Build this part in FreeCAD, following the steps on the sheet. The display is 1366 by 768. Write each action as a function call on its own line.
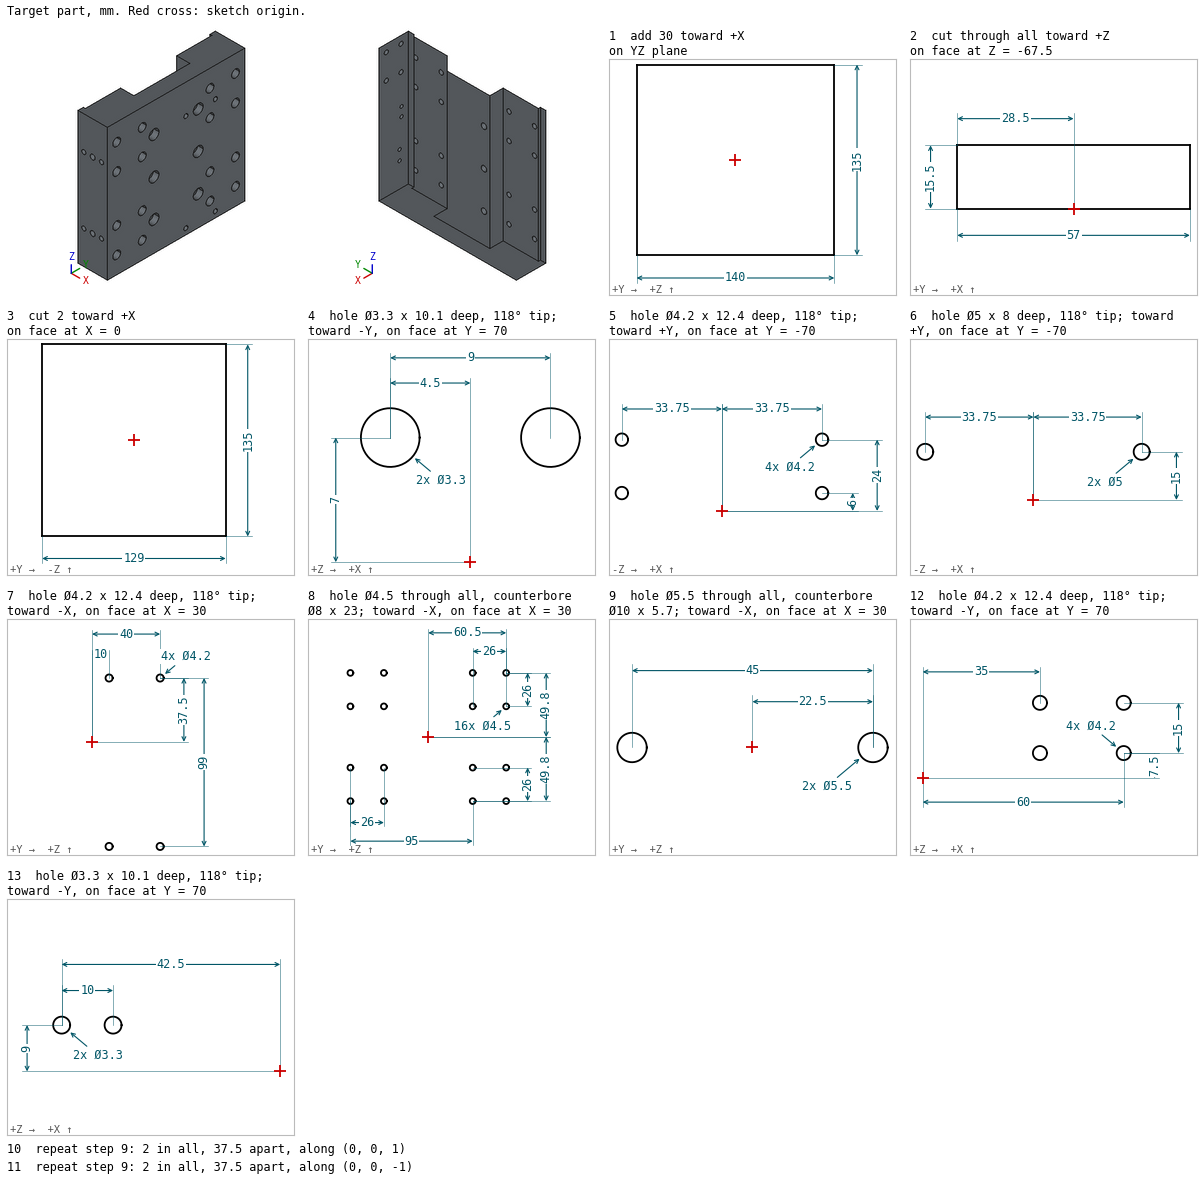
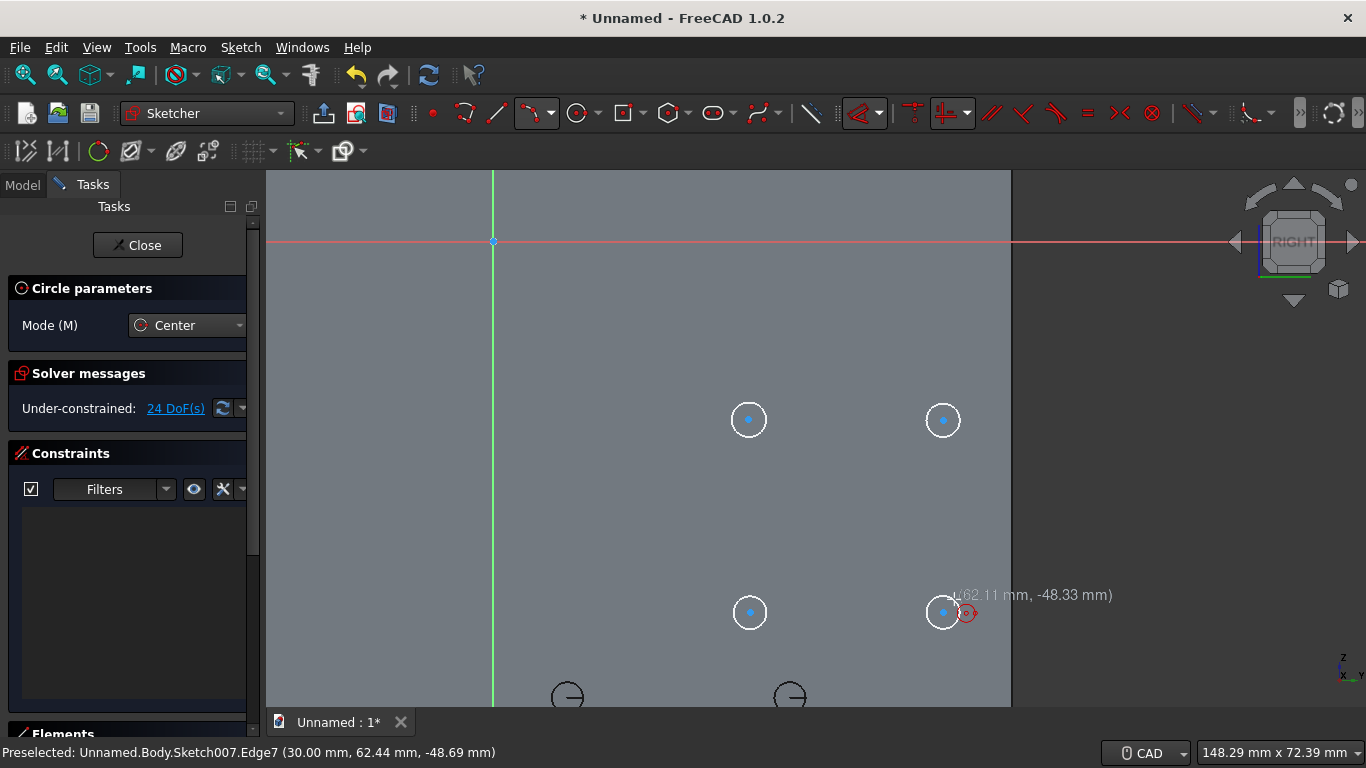
scroll(955, 599, down, 4)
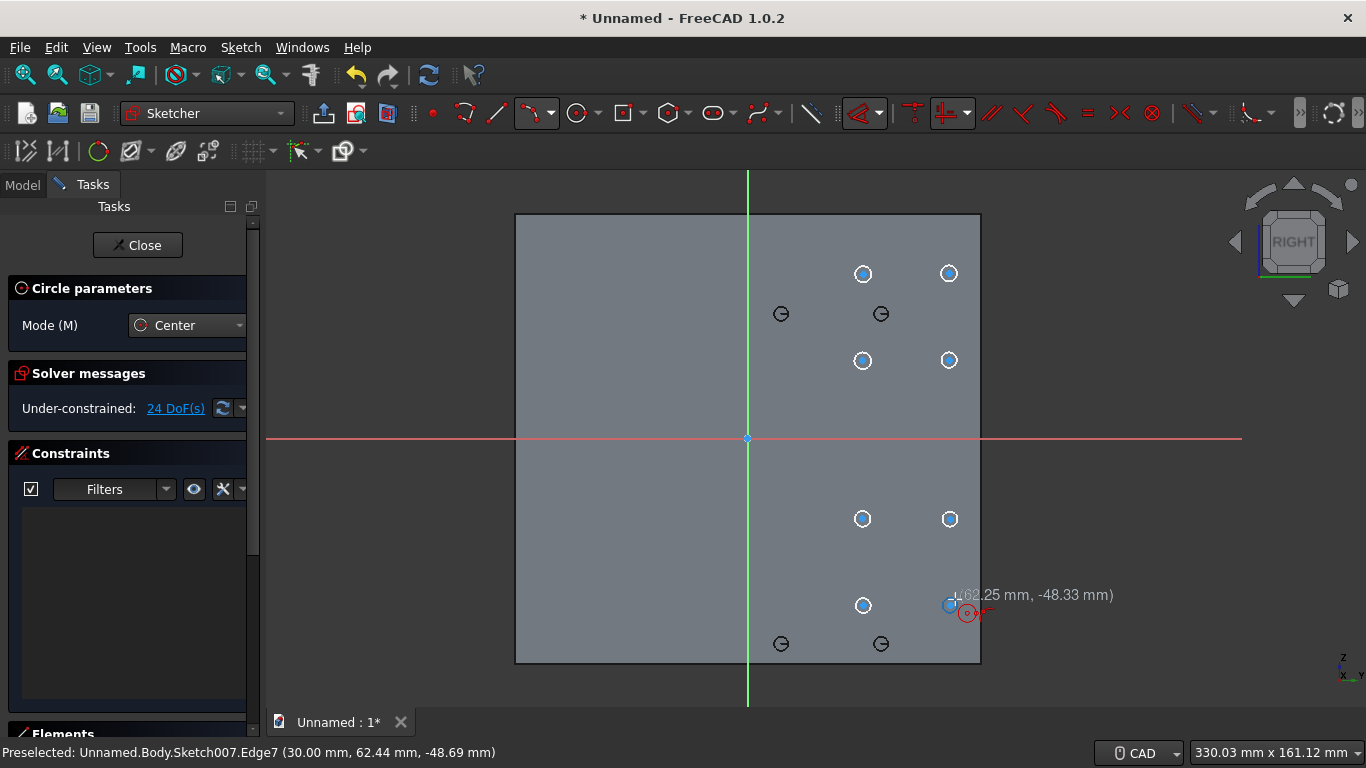
scroll(546, 605, up, 6)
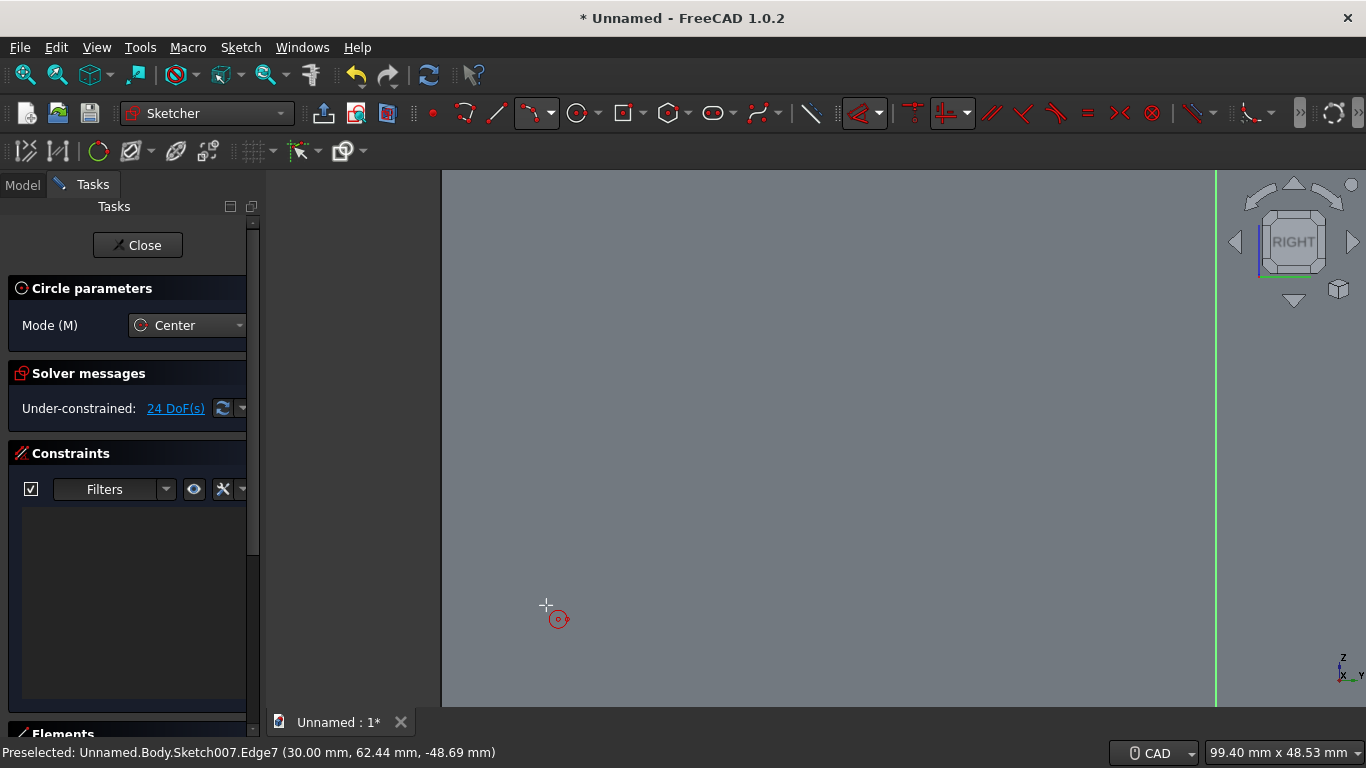
scroll(546, 605, down, 6)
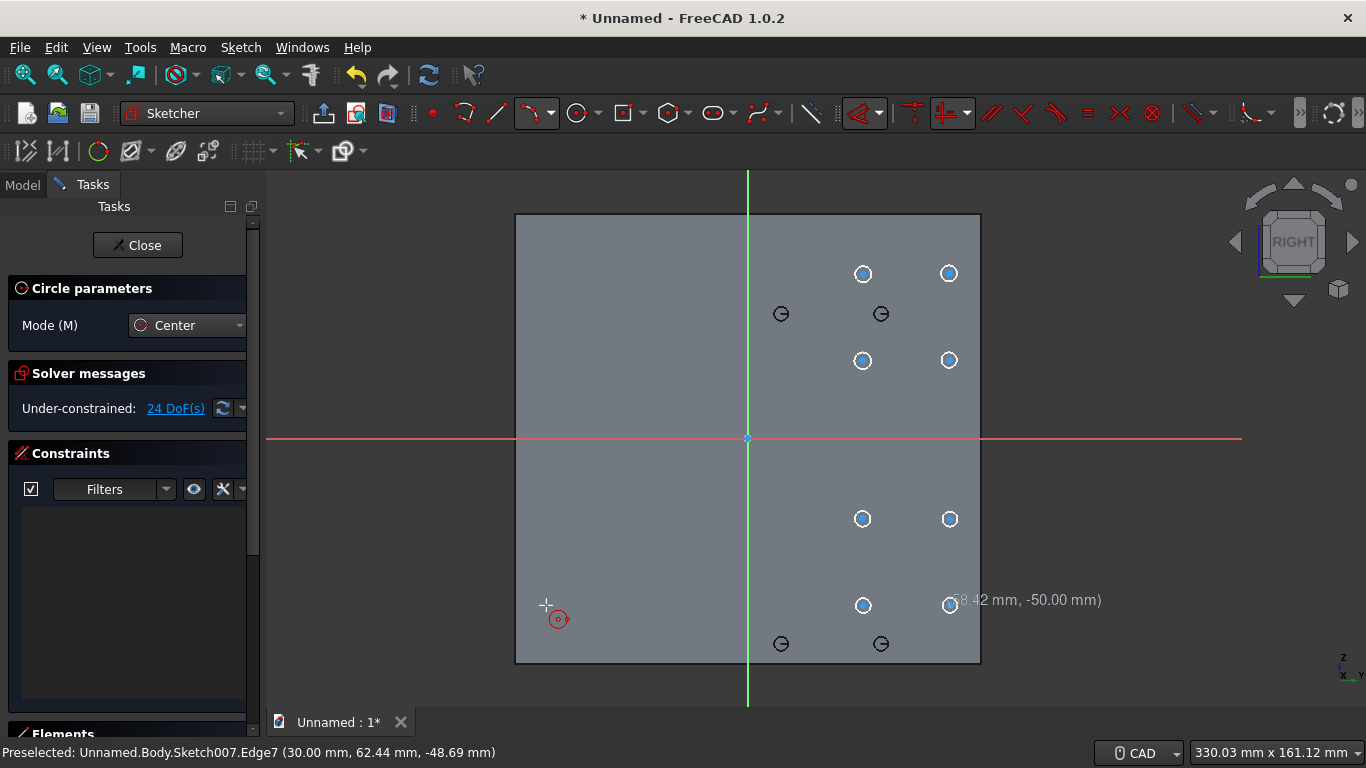
click(546, 605)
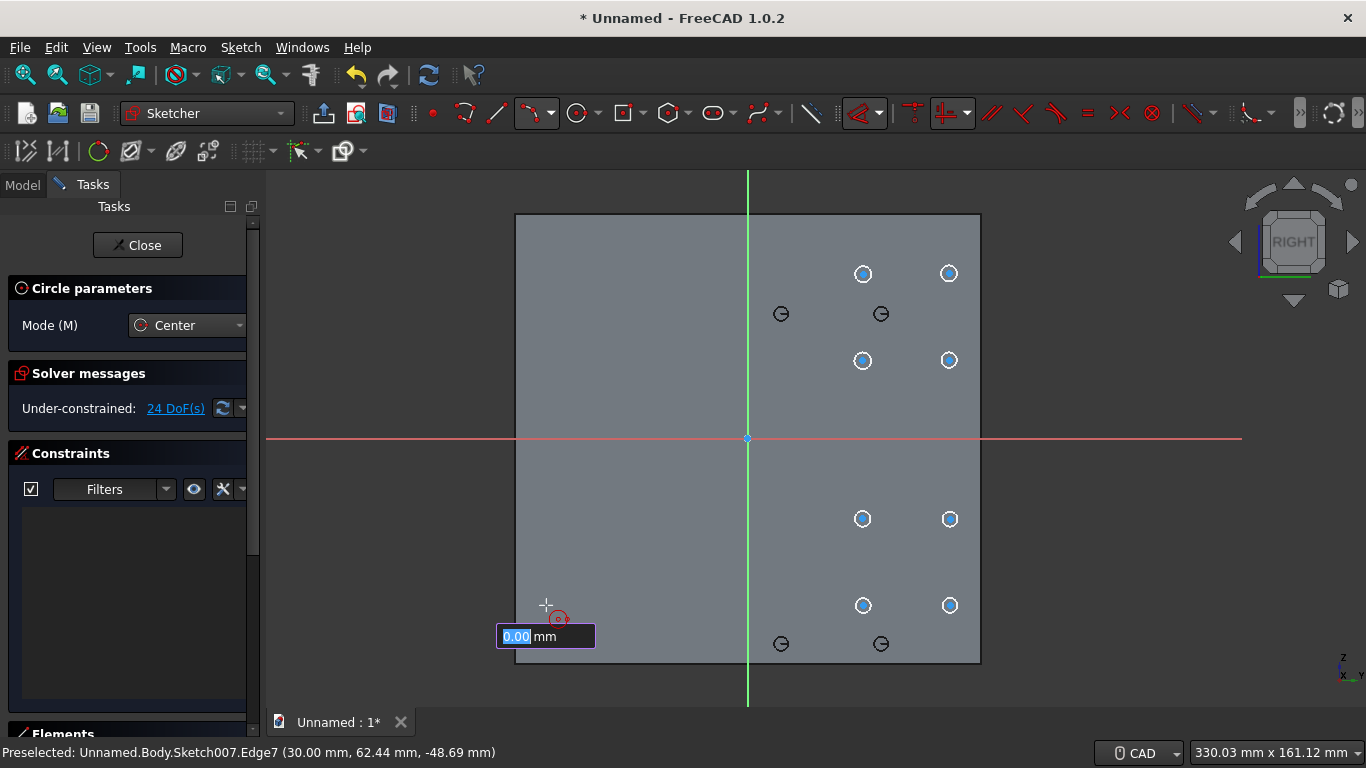
scroll(552, 599, up, 4)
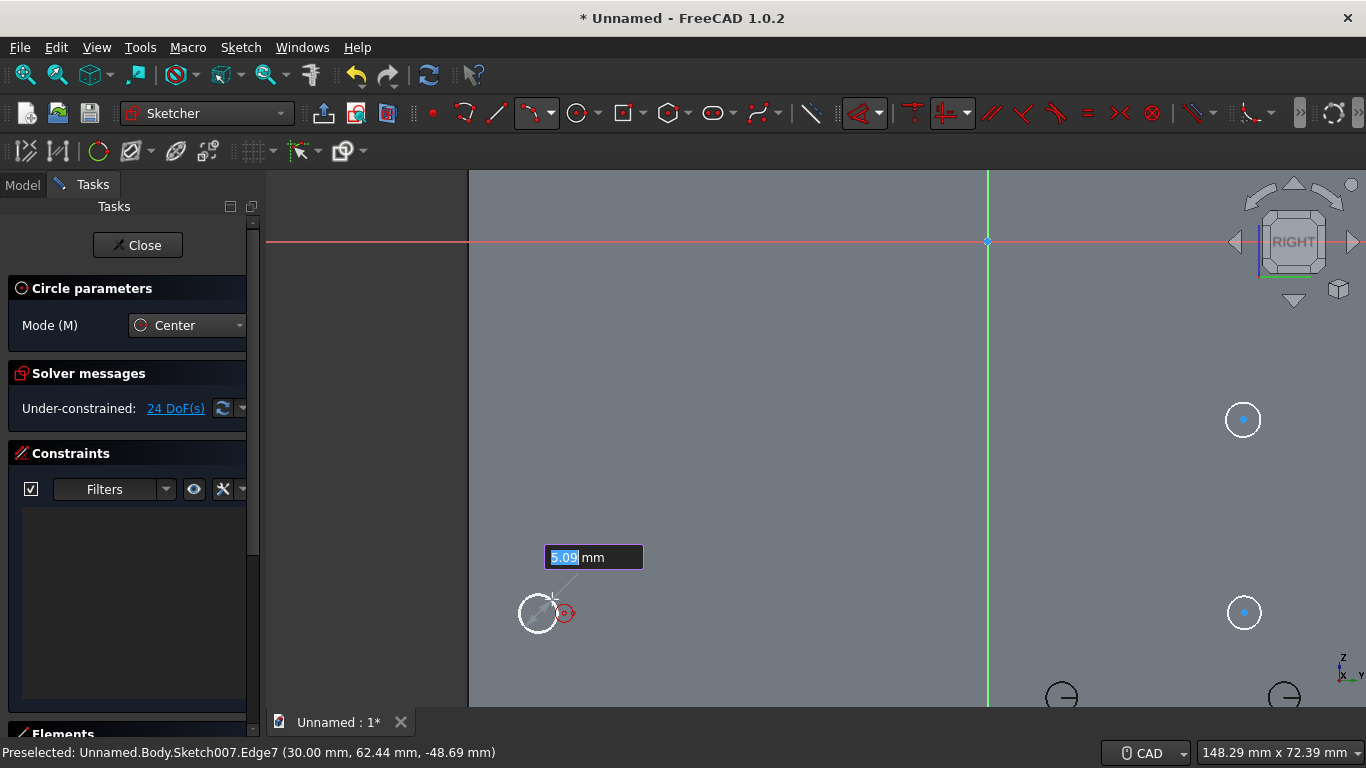
click(551, 599)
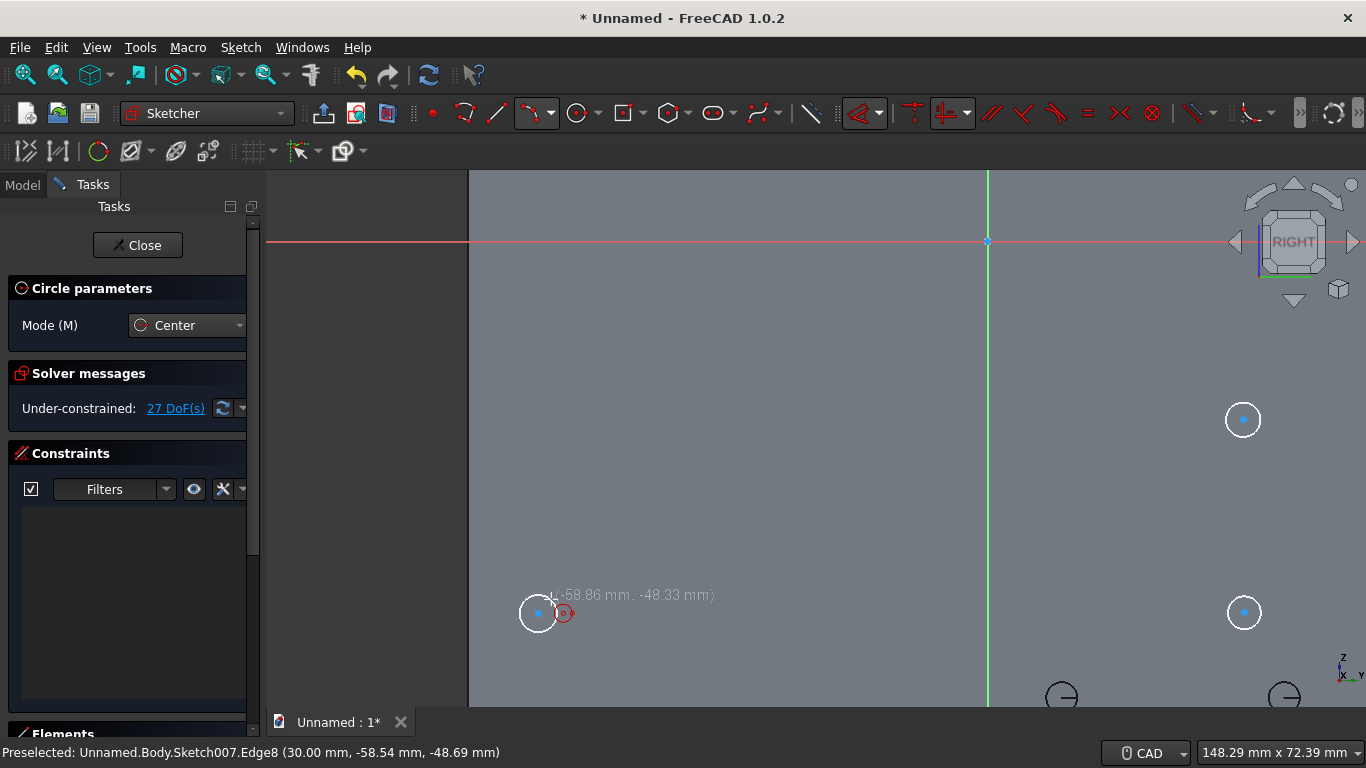
scroll(539, 418, up, 2)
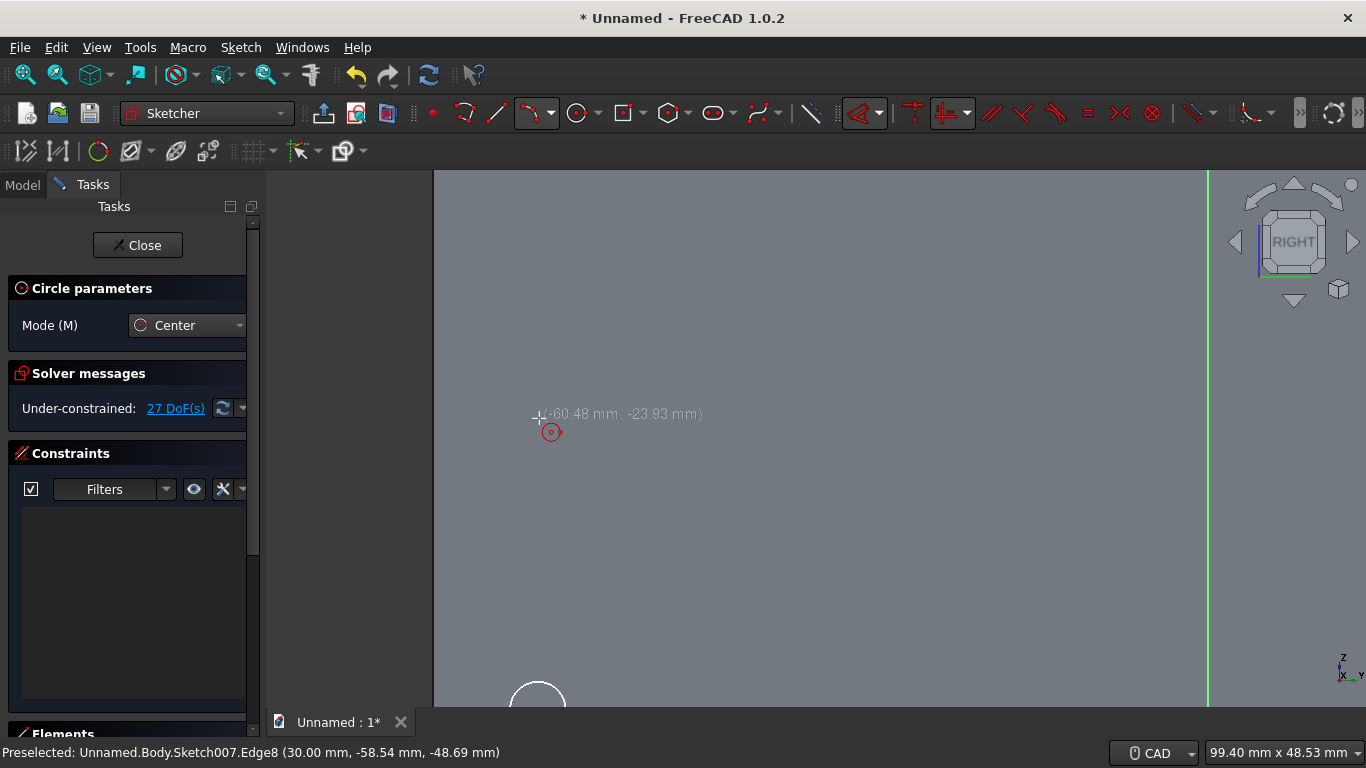
scroll(549, 561, down, 6)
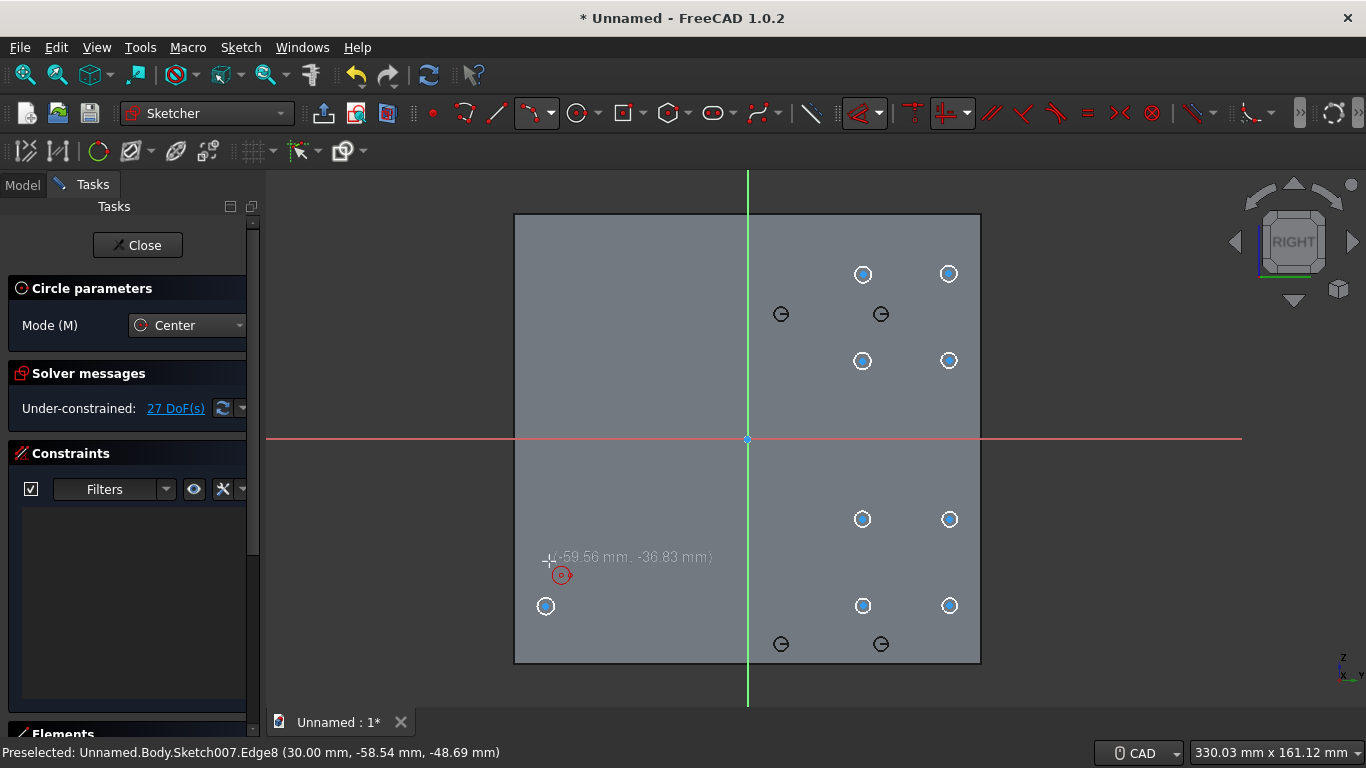
click(546, 518)